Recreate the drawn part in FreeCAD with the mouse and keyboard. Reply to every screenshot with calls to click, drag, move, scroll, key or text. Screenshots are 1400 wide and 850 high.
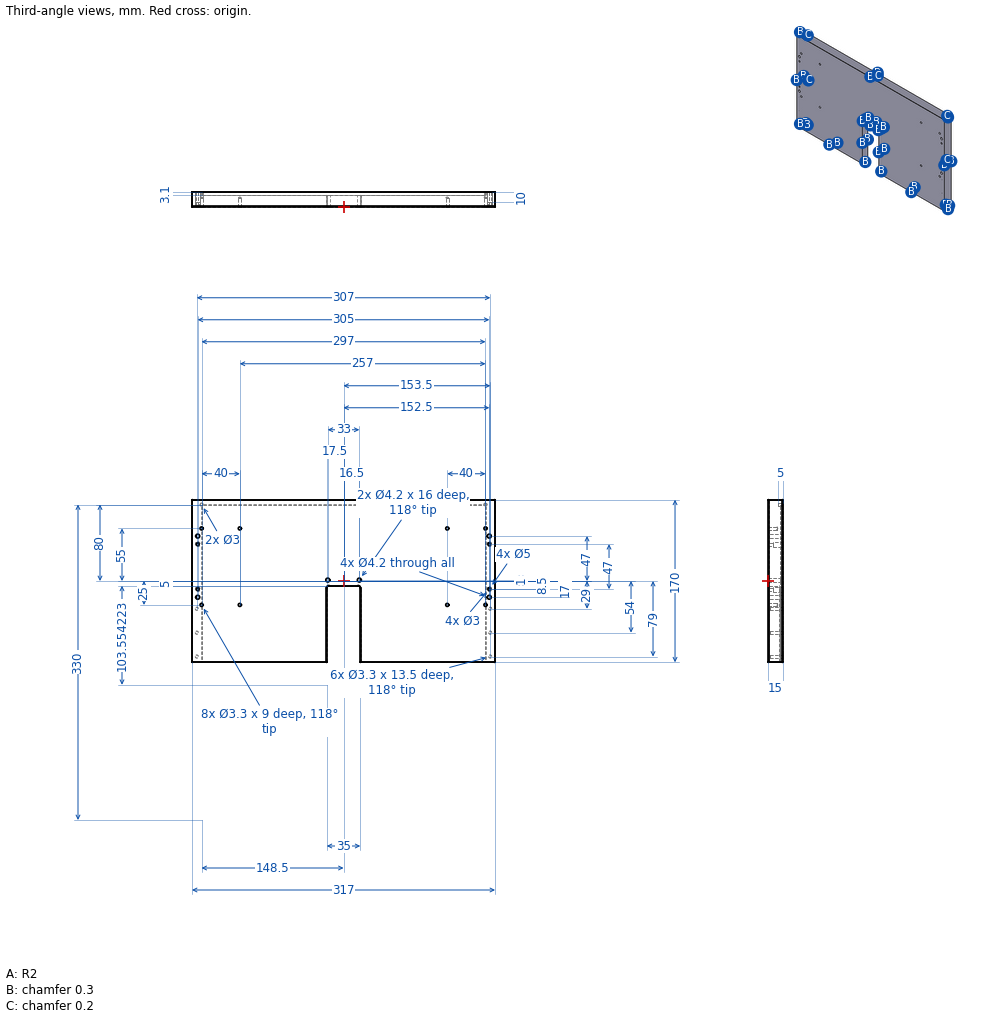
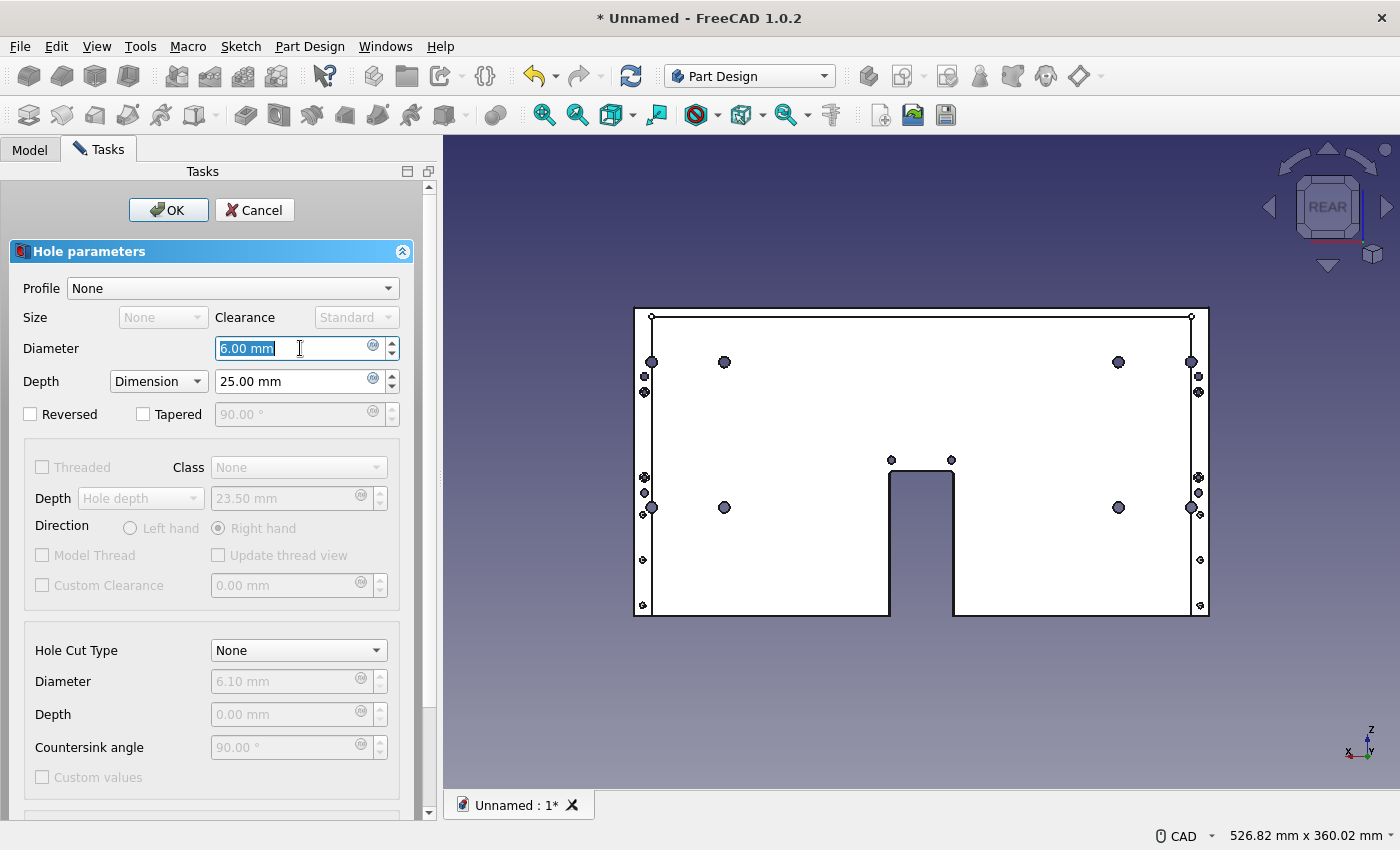
text(3.3)
key(Tab)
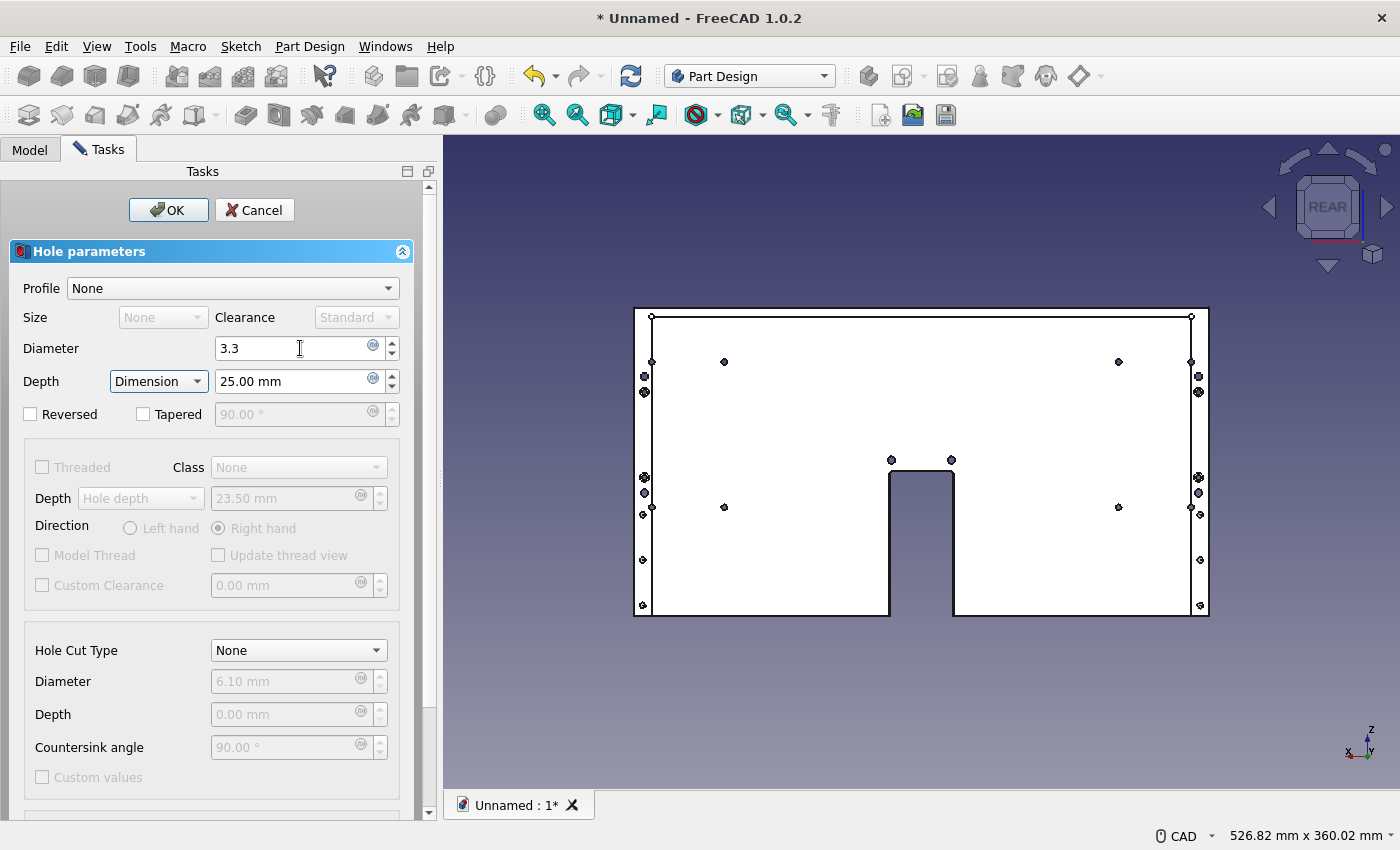
triple_click(300, 382)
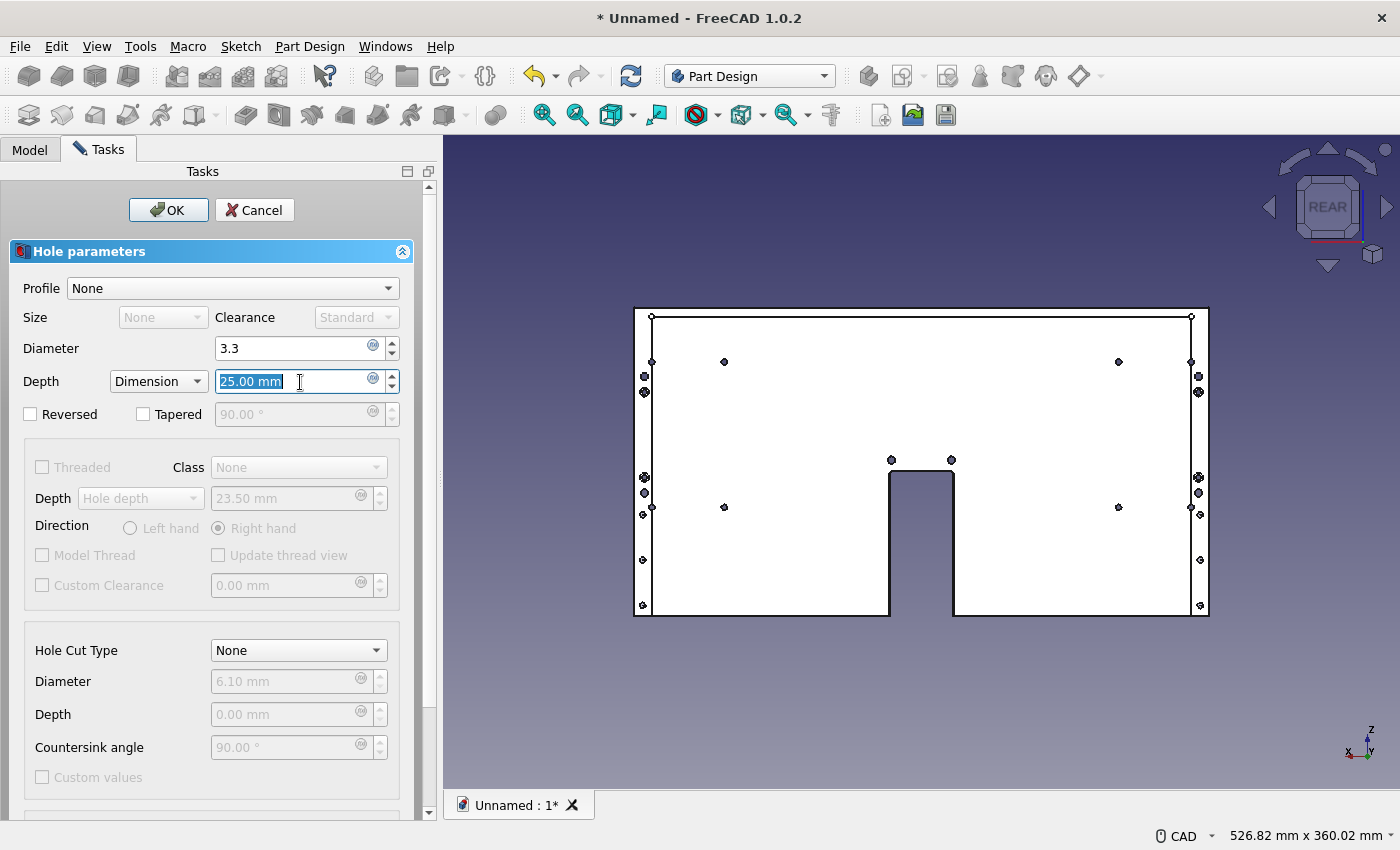
text(9)
key(Tab)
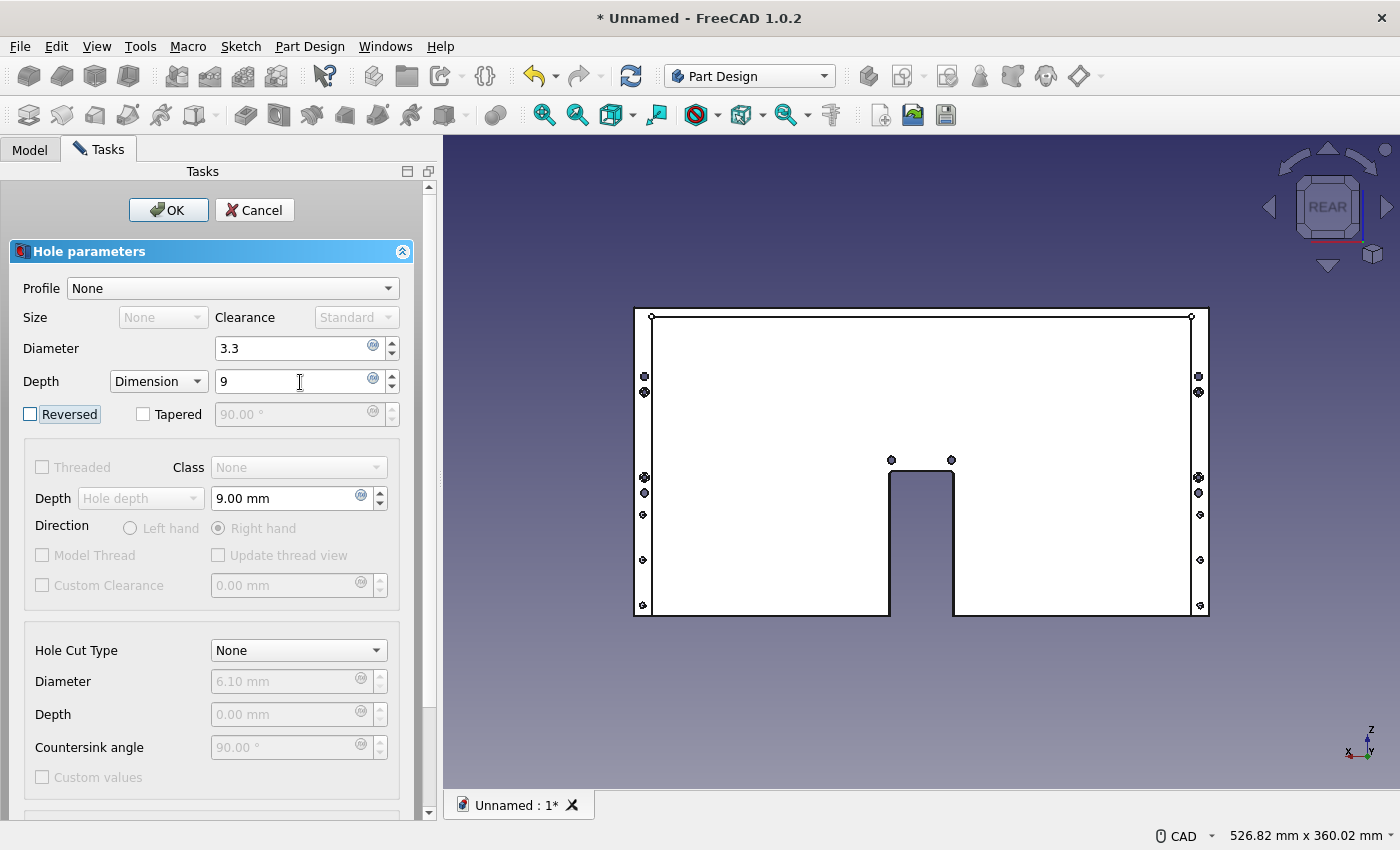
click(169, 210)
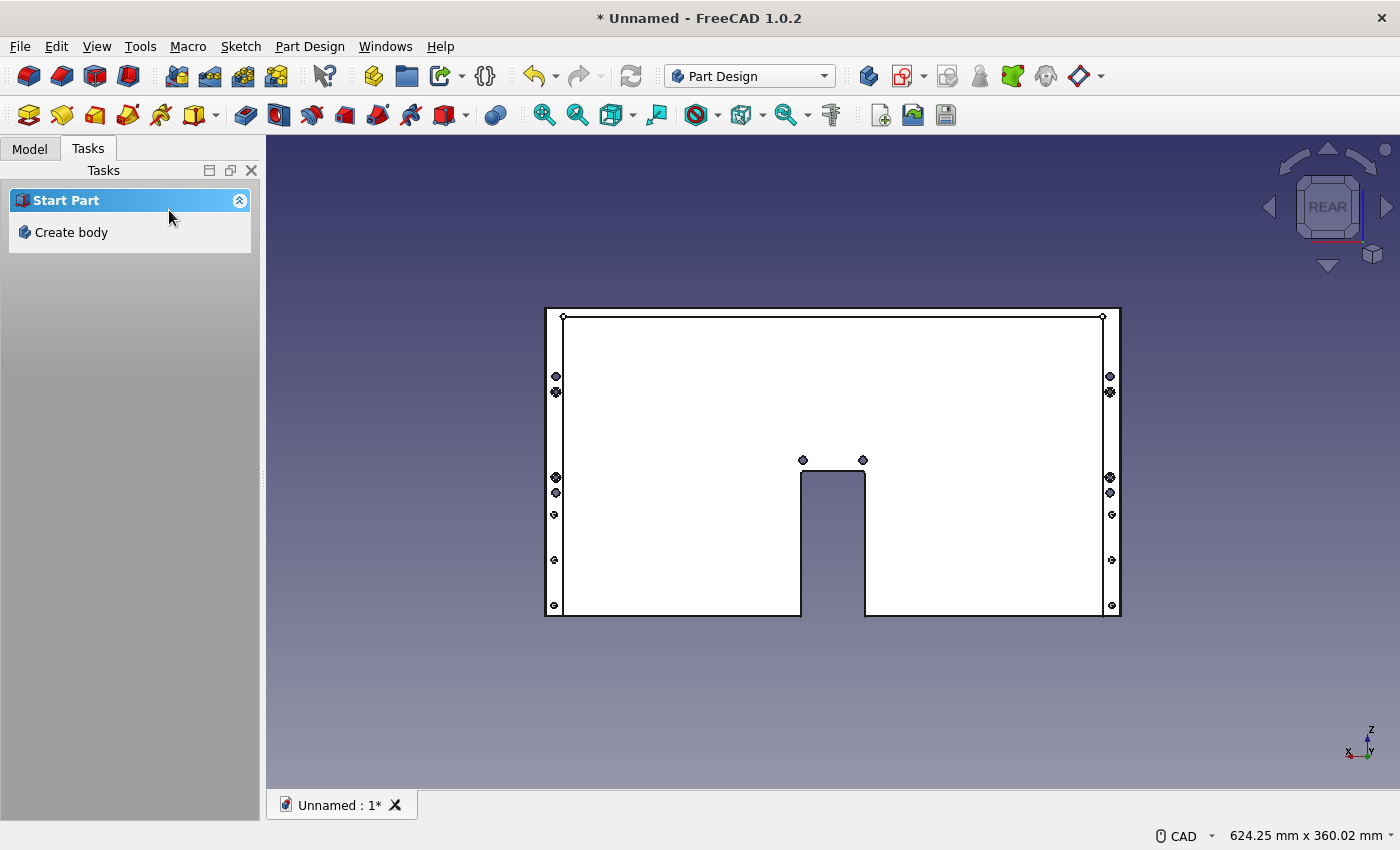
click(563, 467)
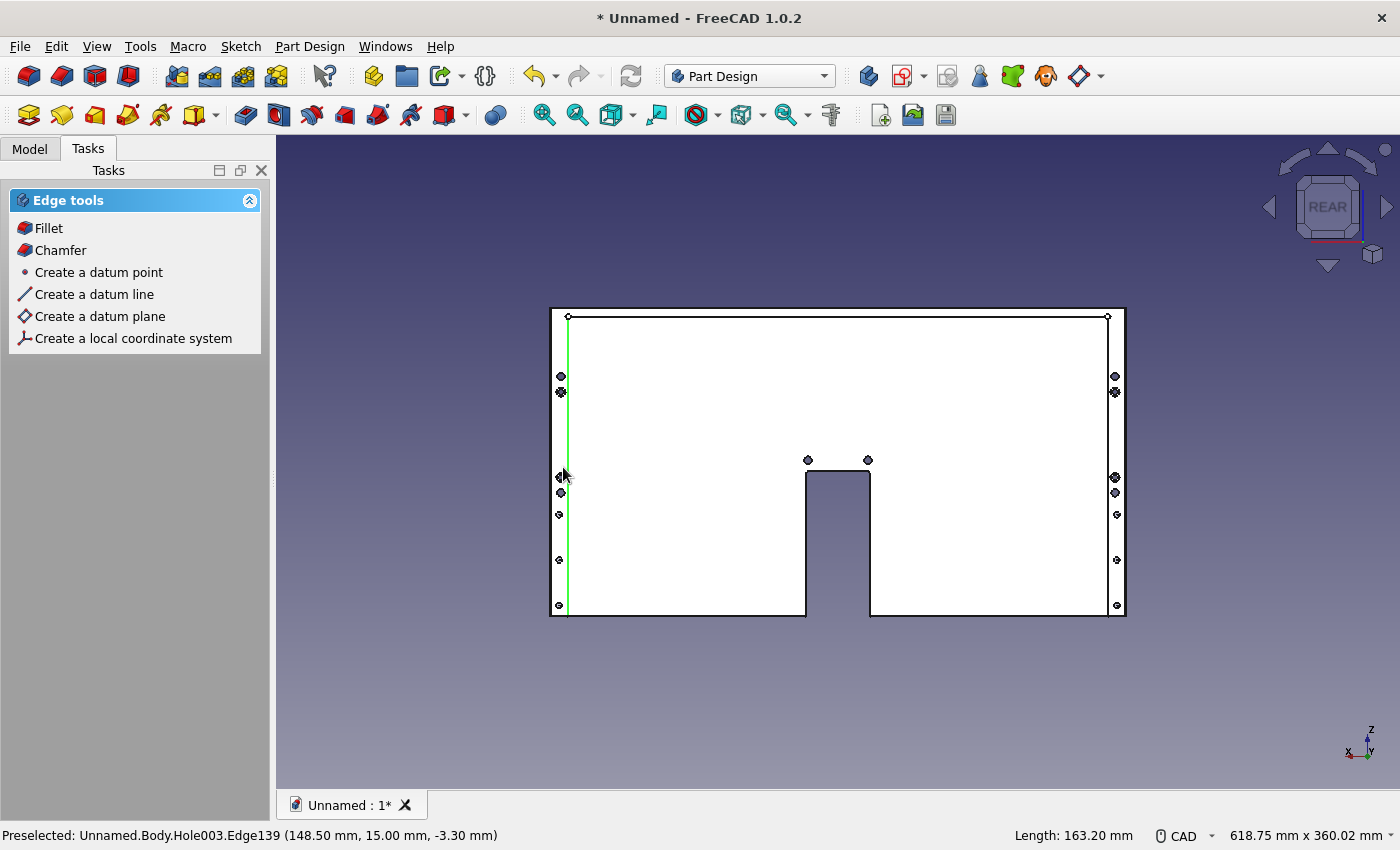
click(838, 316, ctrl)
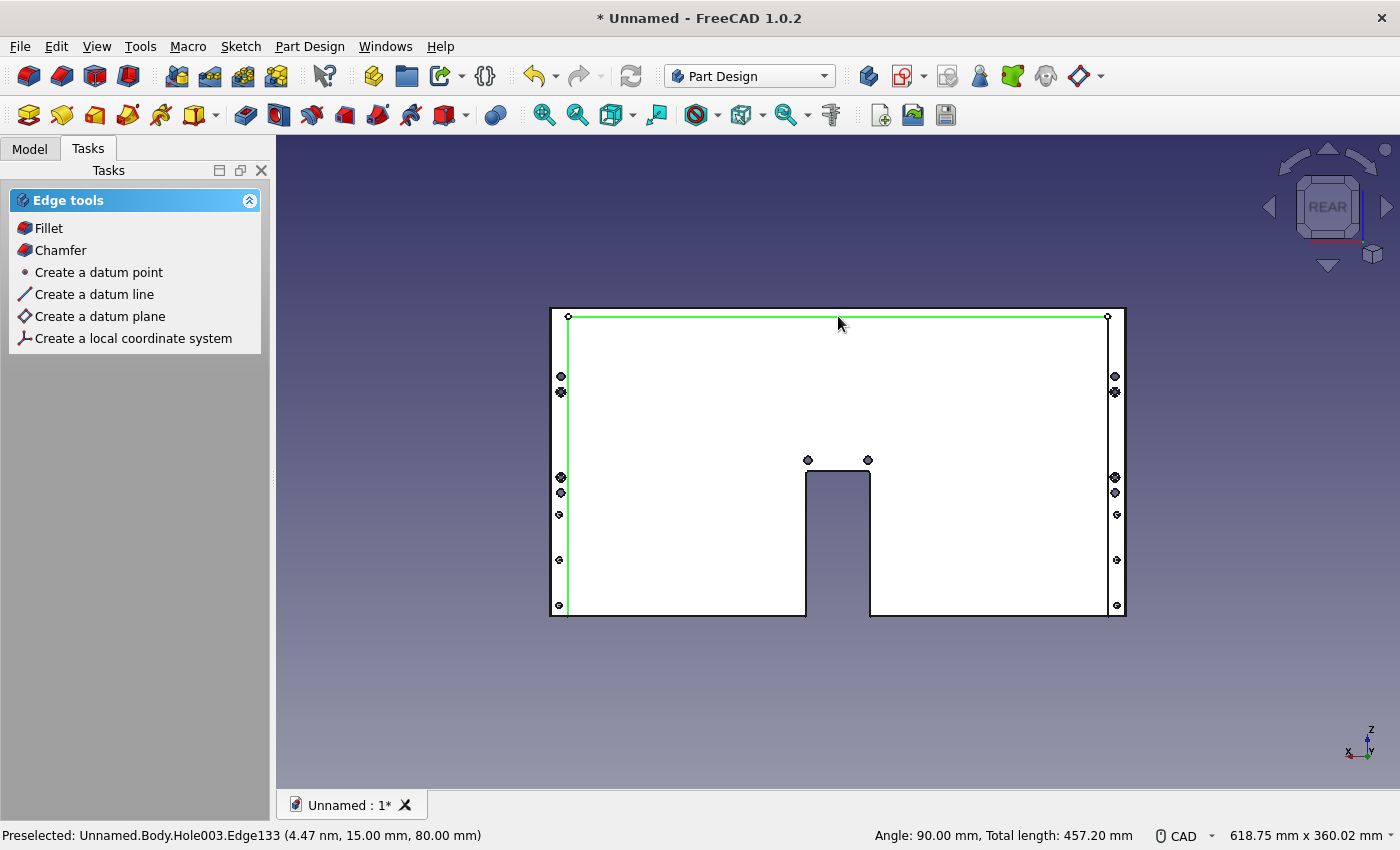
click(1110, 314, ctrl)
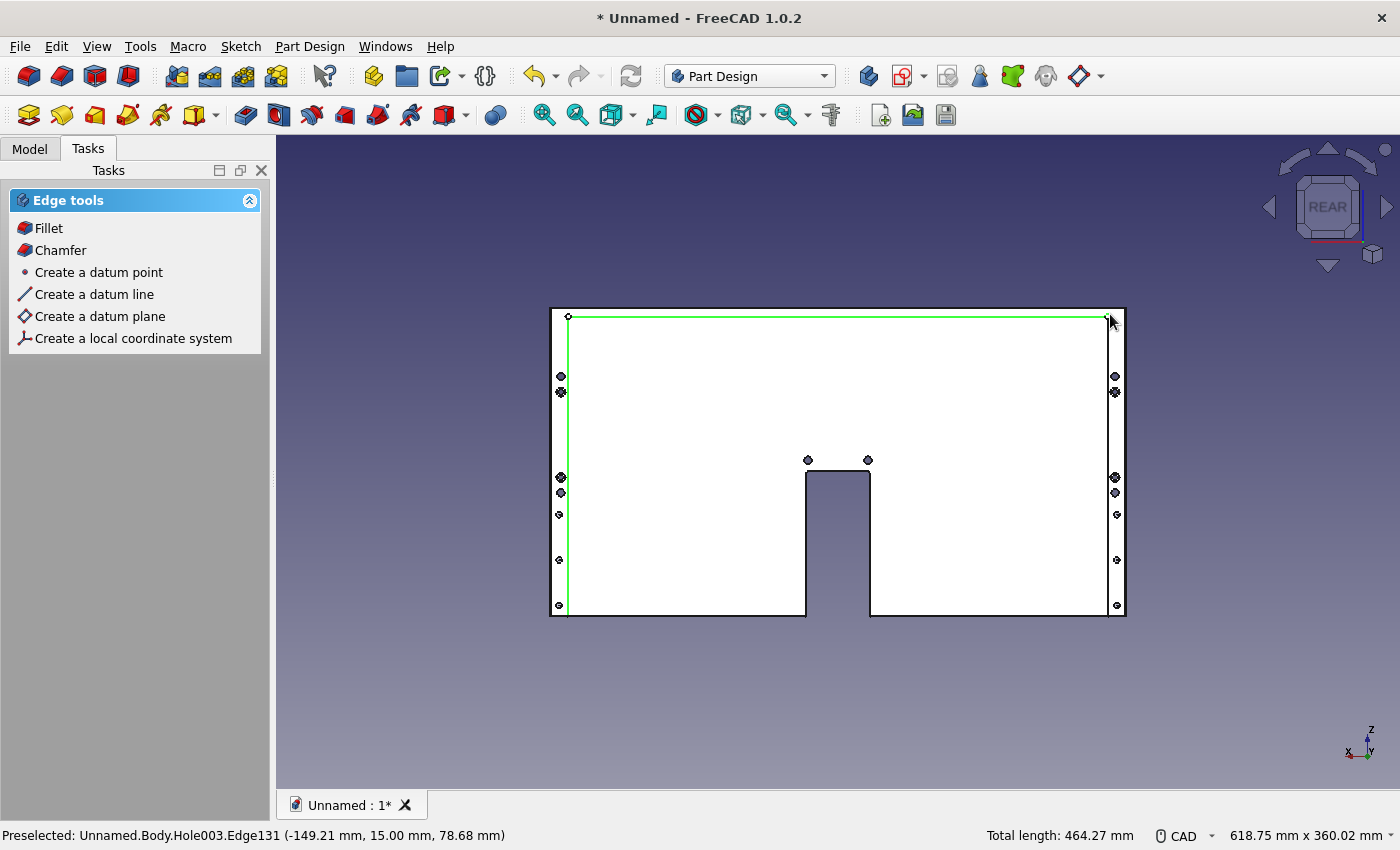
scroll(568, 313, up, 8)